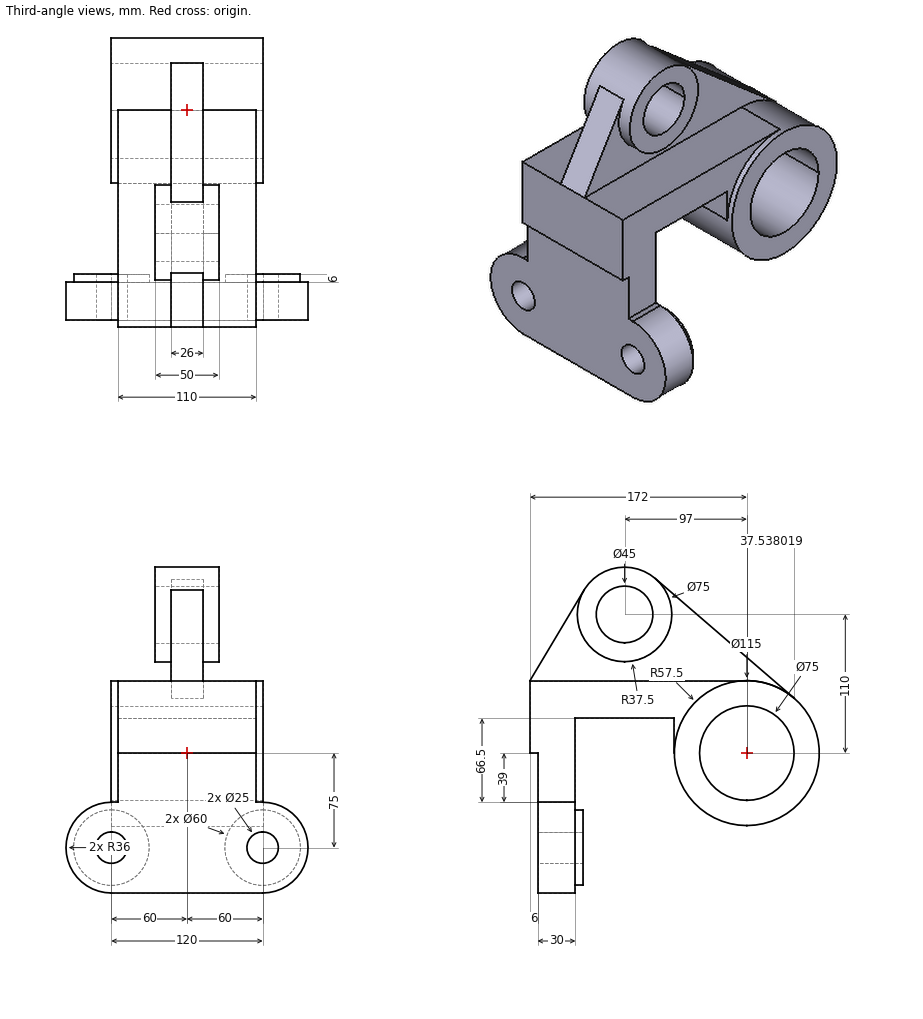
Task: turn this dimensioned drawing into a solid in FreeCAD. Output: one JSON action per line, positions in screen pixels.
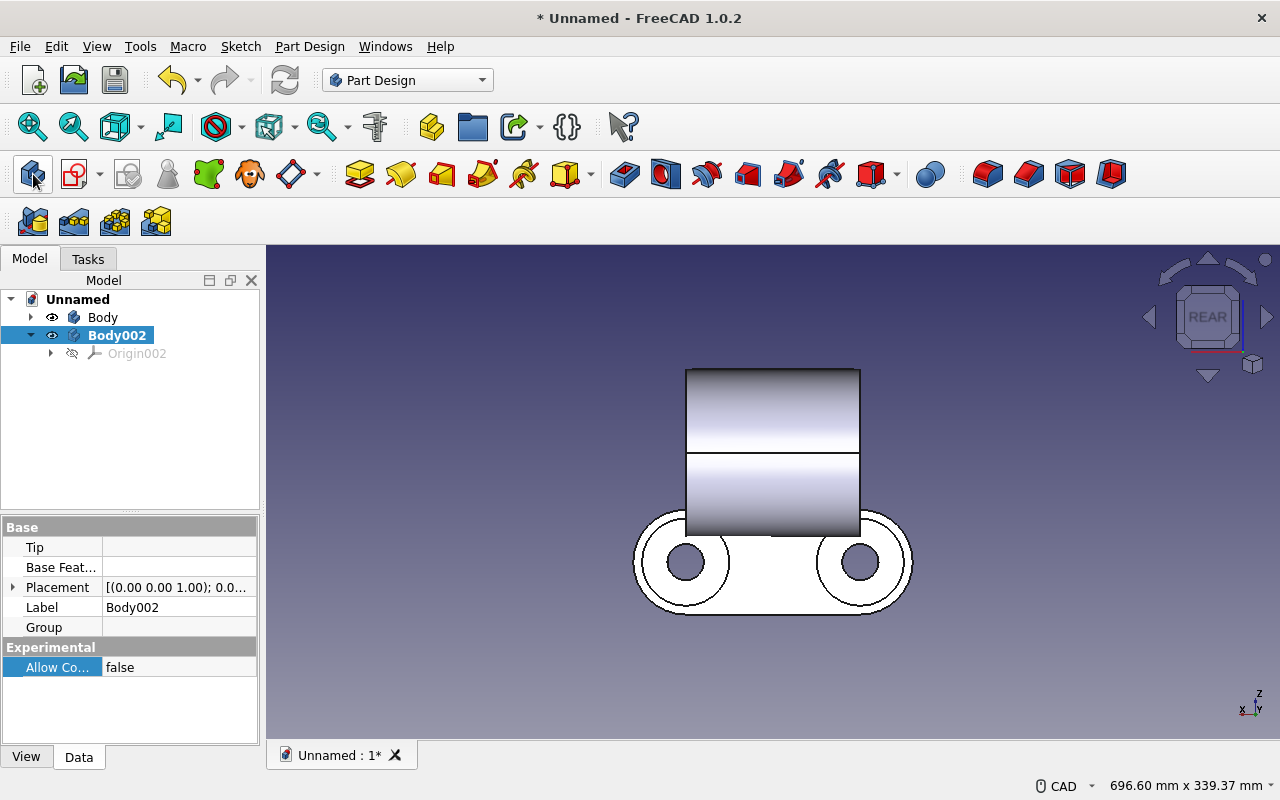
{"action": "left_click", "coordinate": [306, 699]}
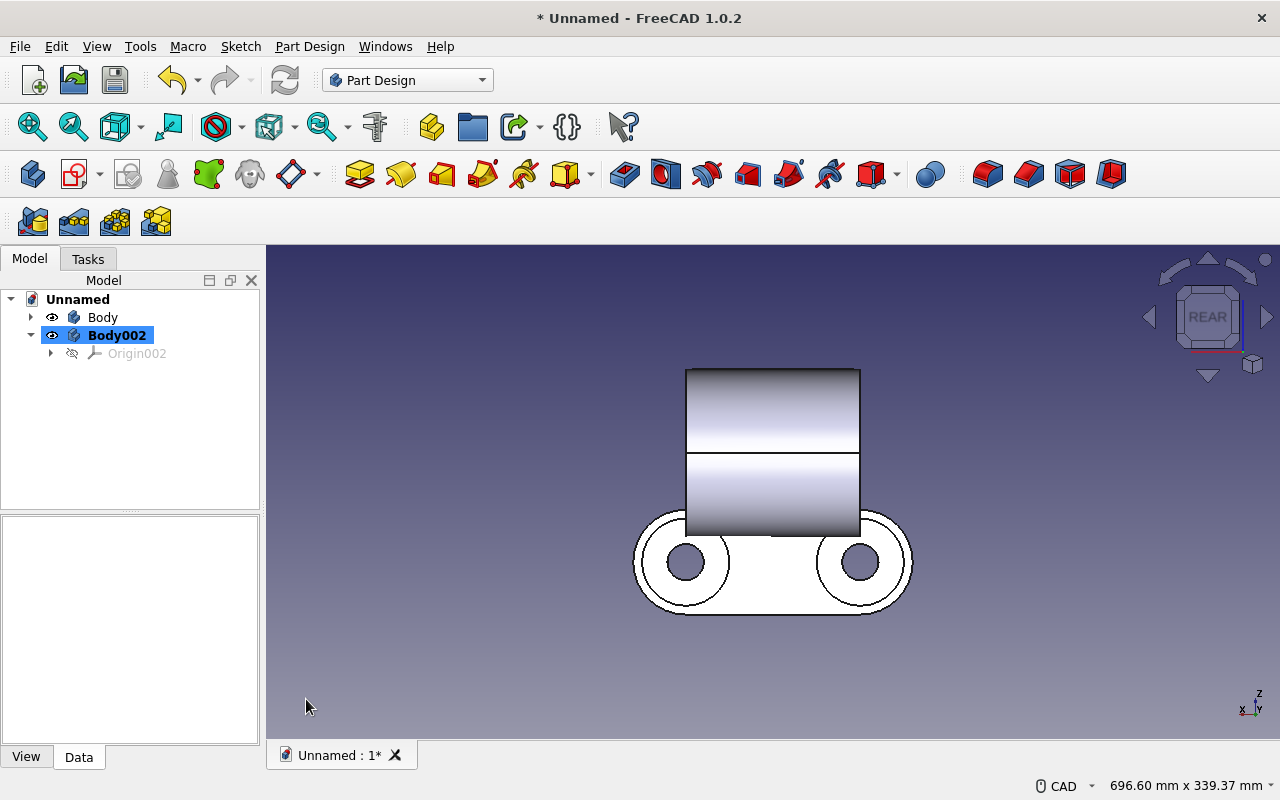
{"action": "left_click", "coordinate": [74, 174]}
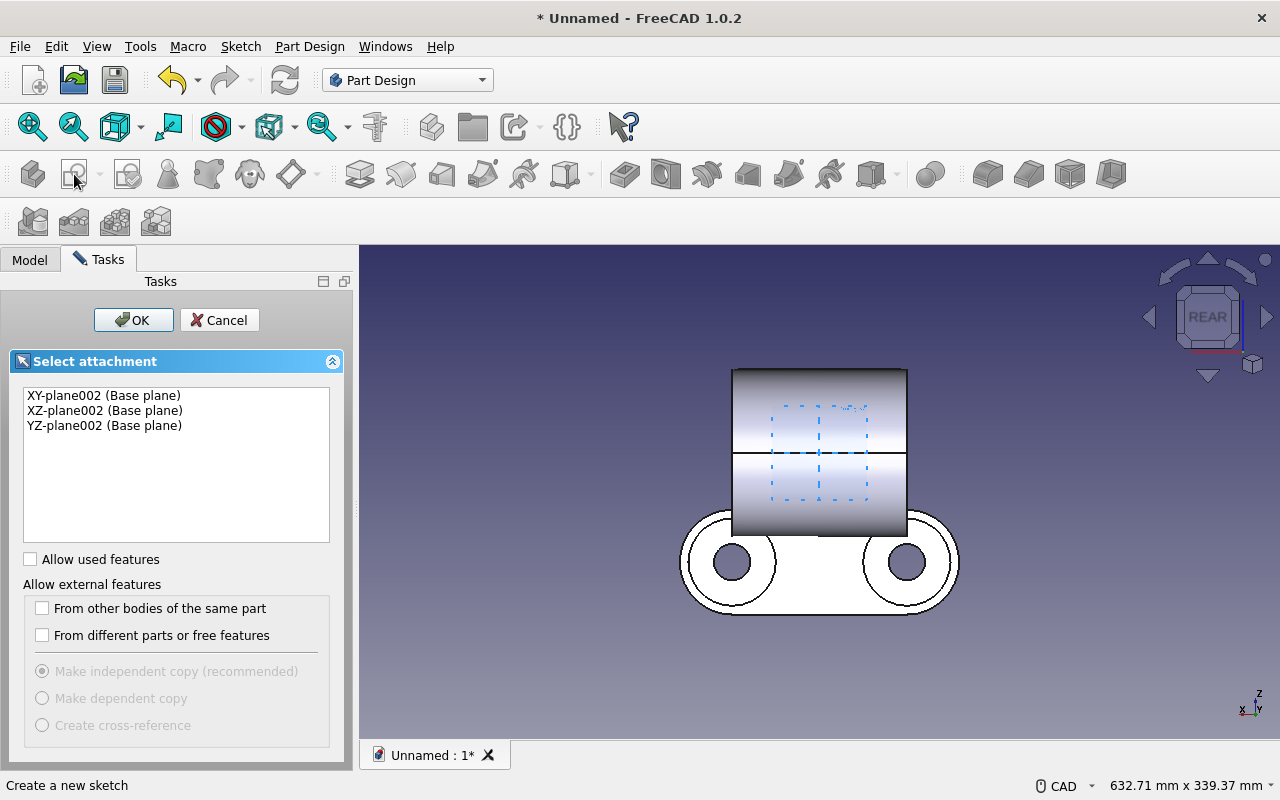
{"action": "left_click", "coordinate": [84, 426]}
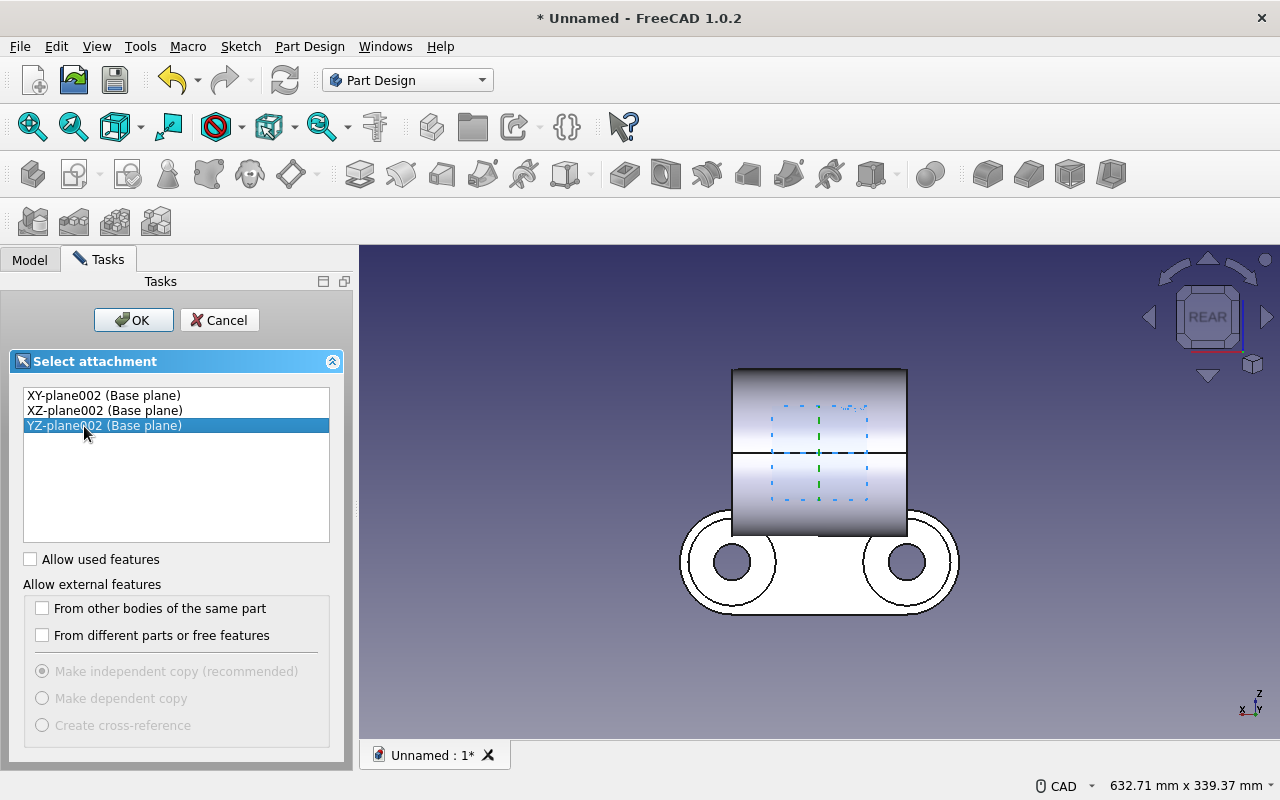
{"action": "left_click", "coordinate": [134, 320]}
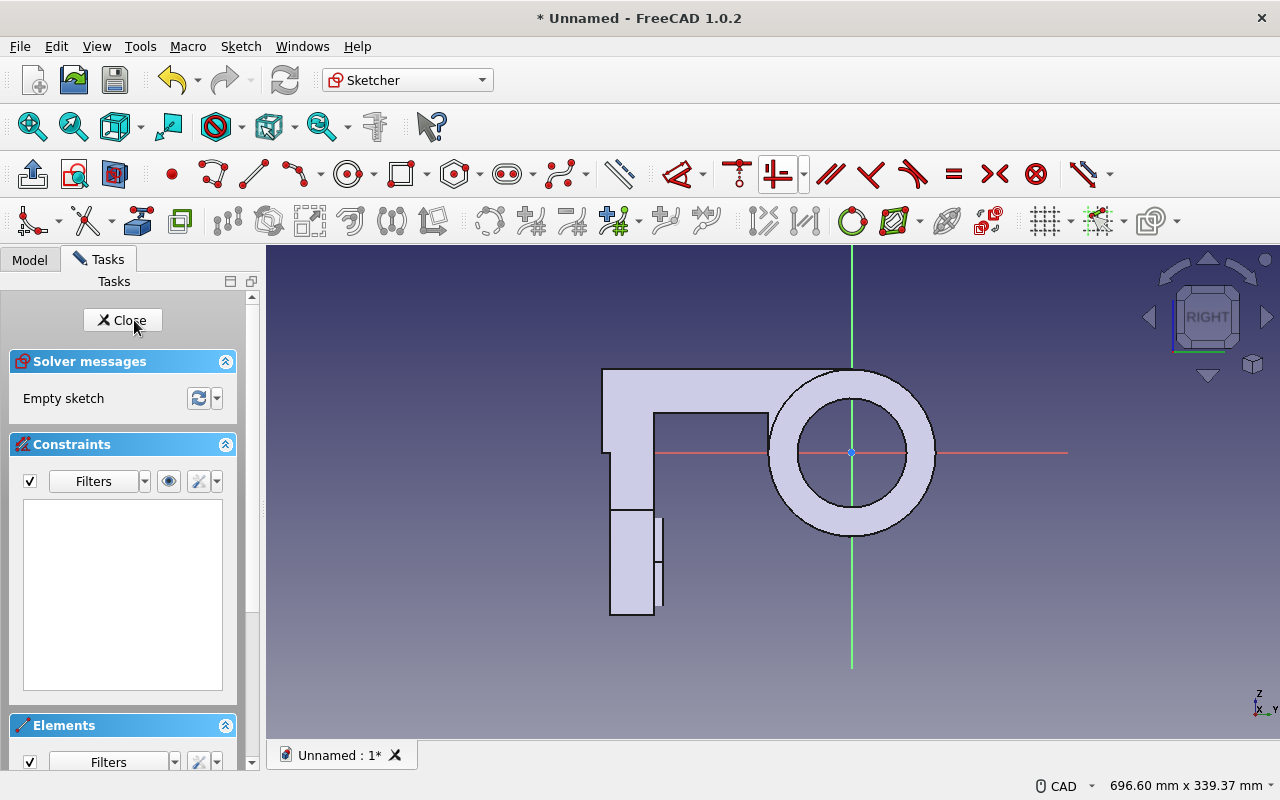
{"action": "scroll", "coordinate": [481, 711], "scroll_direction": "down", "scroll_amount": 1}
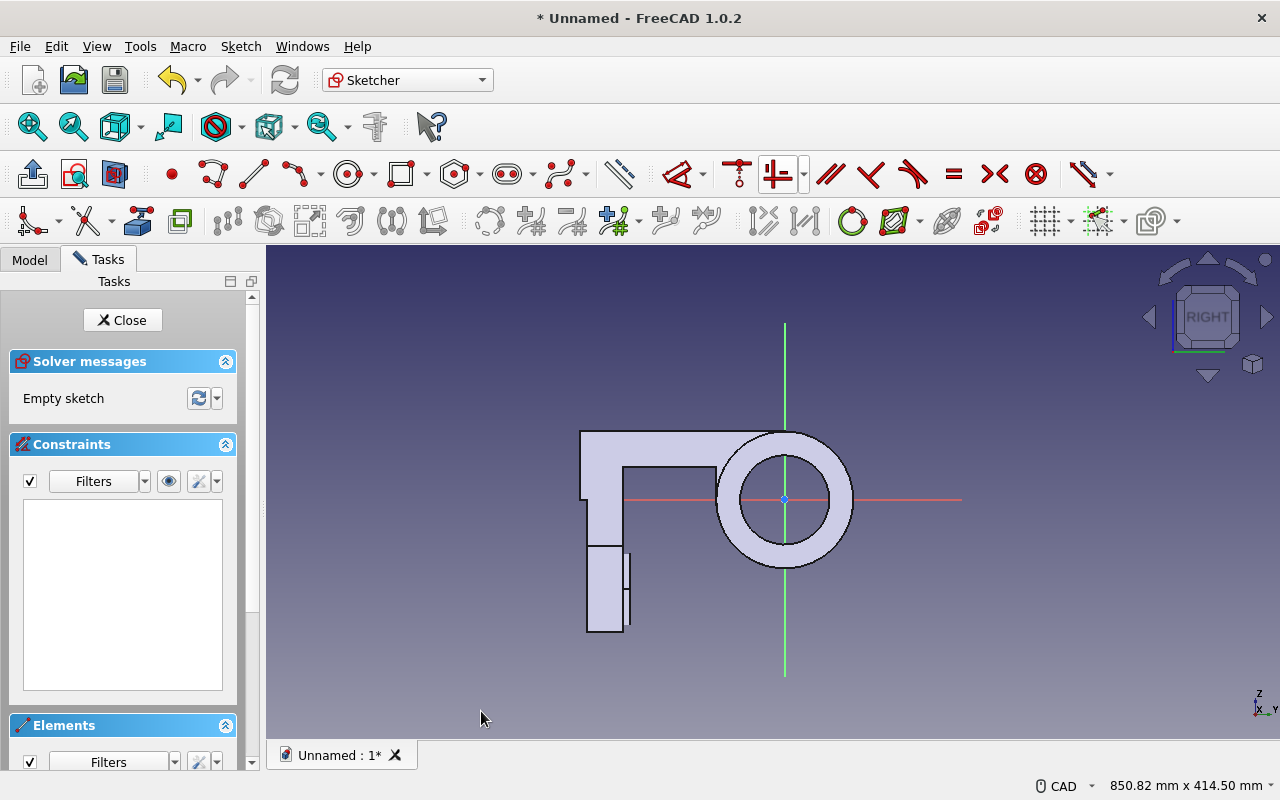
{"action": "scroll", "coordinate": [705, 315], "scroll_direction": "up", "scroll_amount": 3}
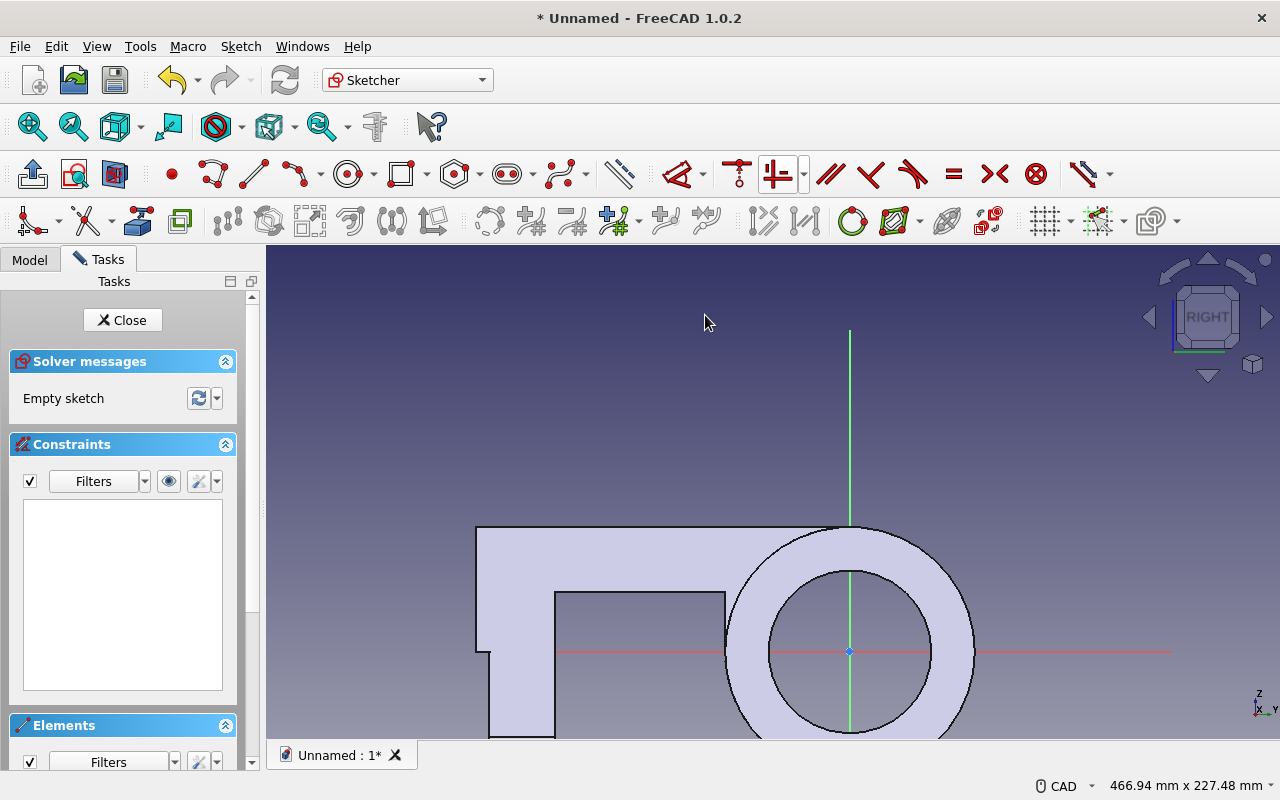
{"action": "key", "text": "g c"}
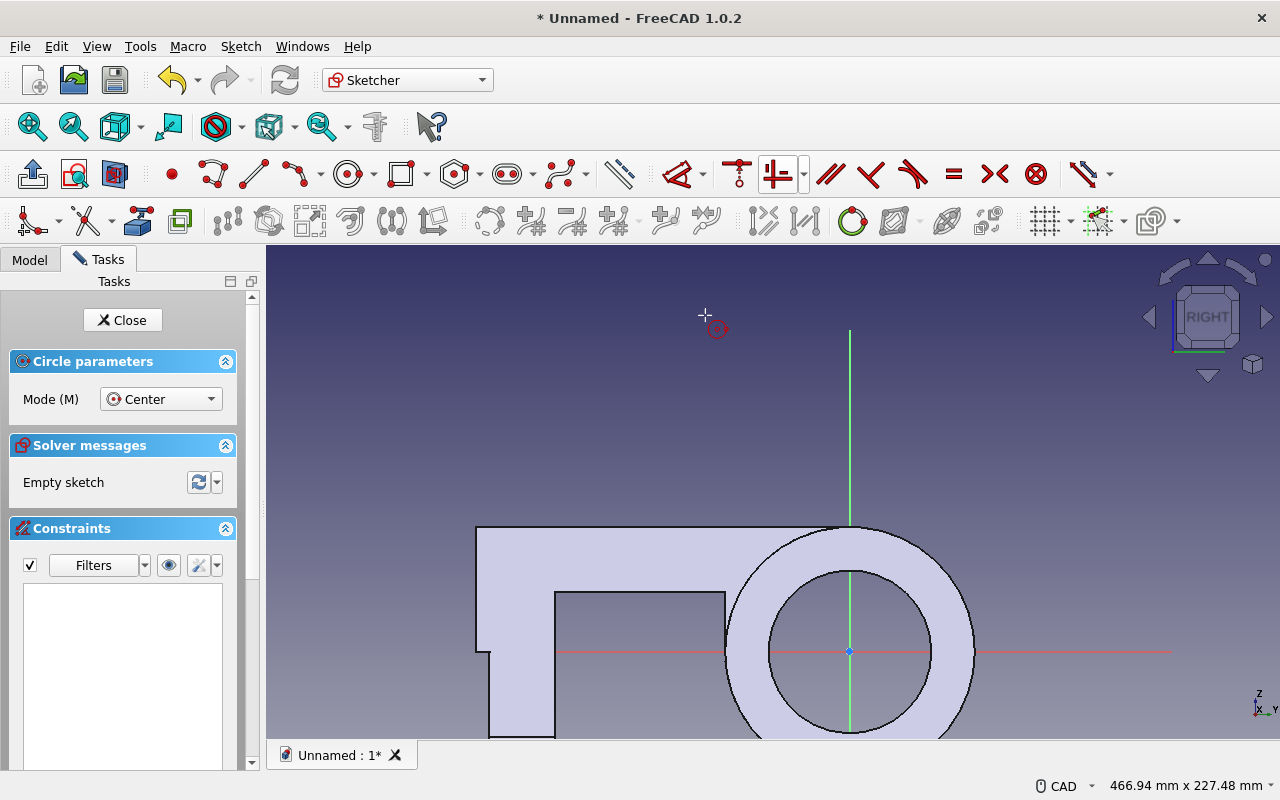
{"action": "left_click", "coordinate": [639, 413]}
{"action": "left_click", "coordinate": [697, 355]}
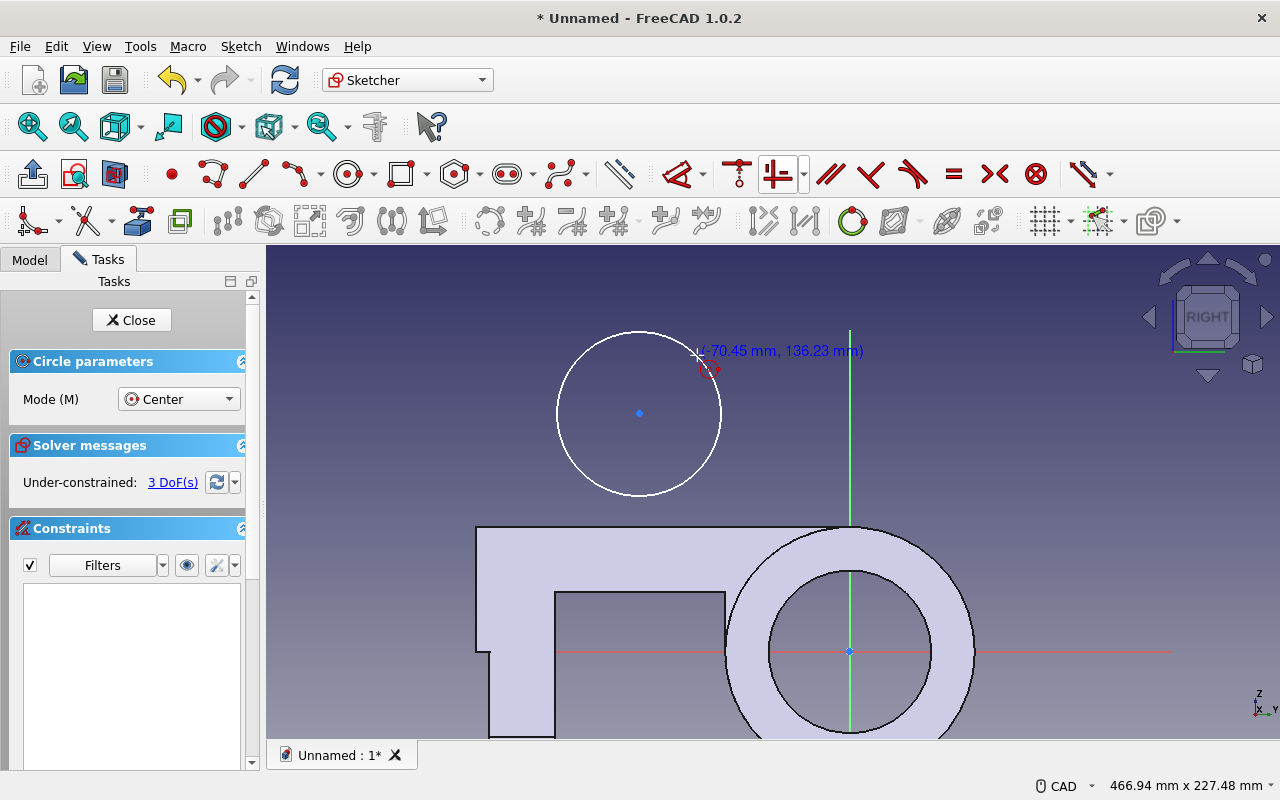
{"action": "left_click", "coordinate": [639, 414]}
{"action": "left_click", "coordinate": [674, 378]}
{"action": "key", "text": "Escape"}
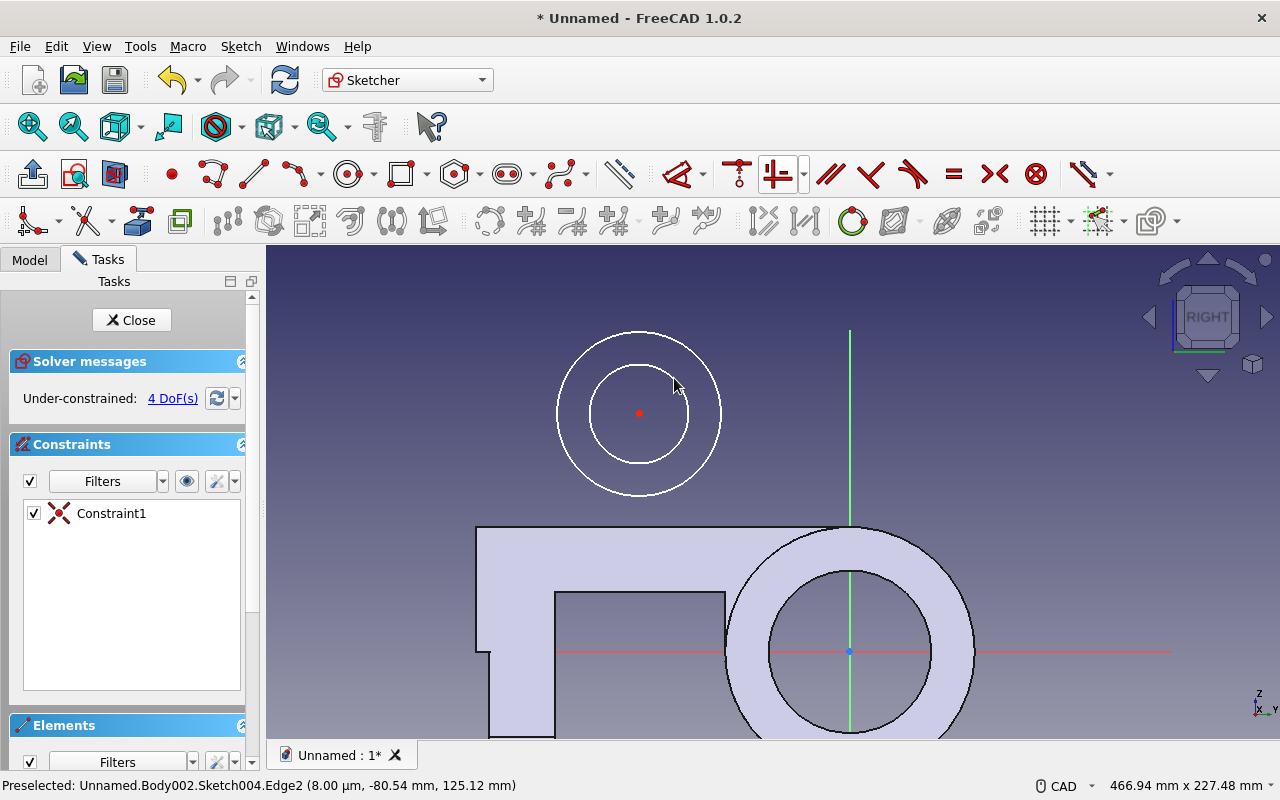
{"action": "left_click", "coordinate": [676, 174]}